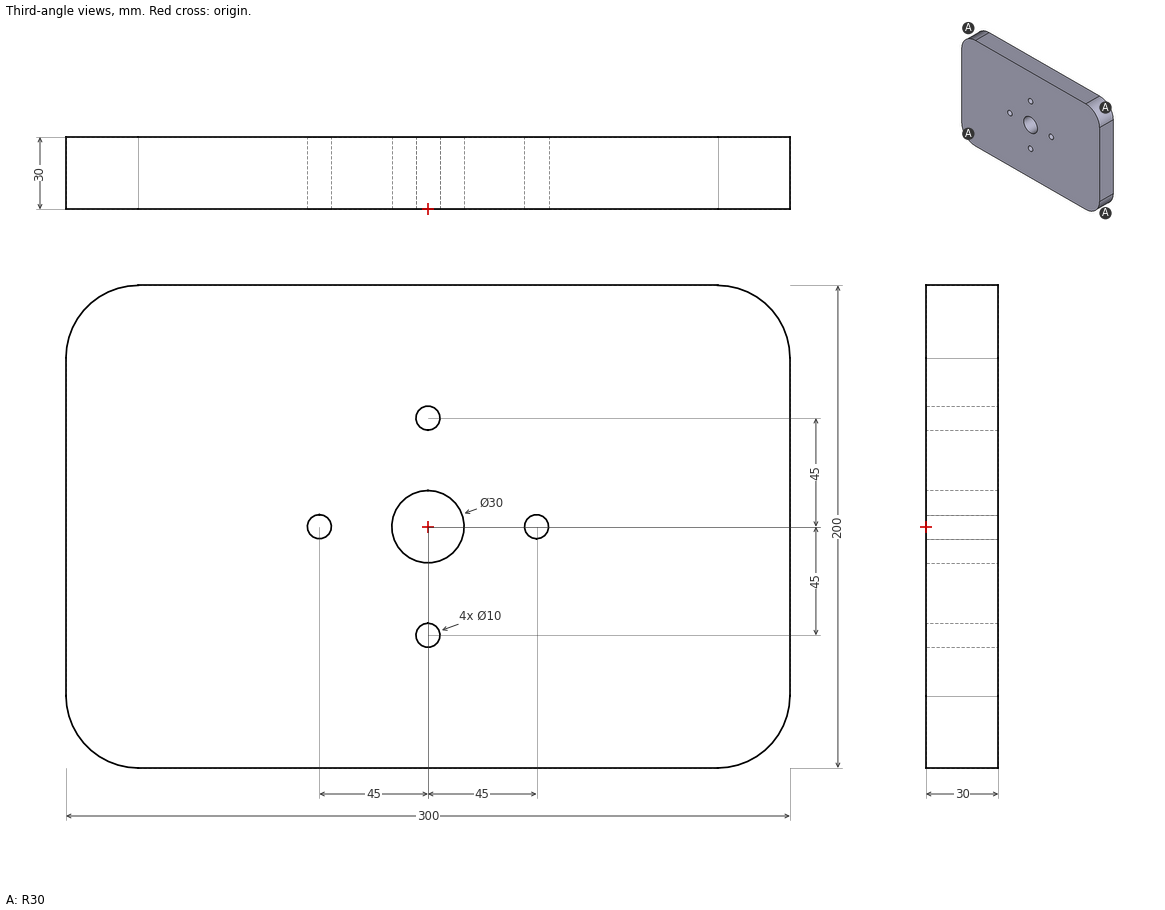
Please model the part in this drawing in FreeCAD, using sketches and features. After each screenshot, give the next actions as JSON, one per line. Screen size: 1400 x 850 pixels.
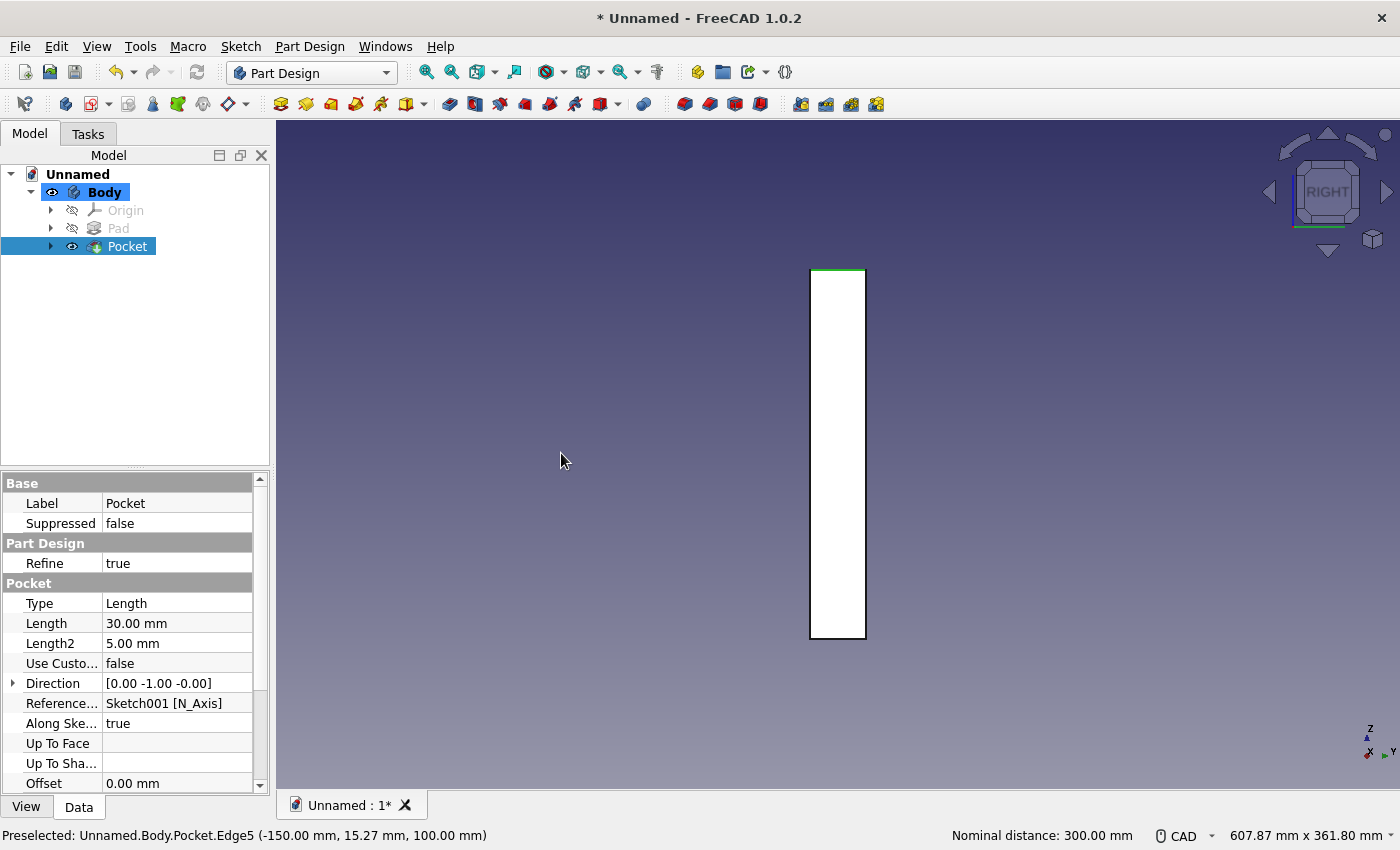
{"action": "left_click", "coordinate": [838, 638], "text": "ctrl"}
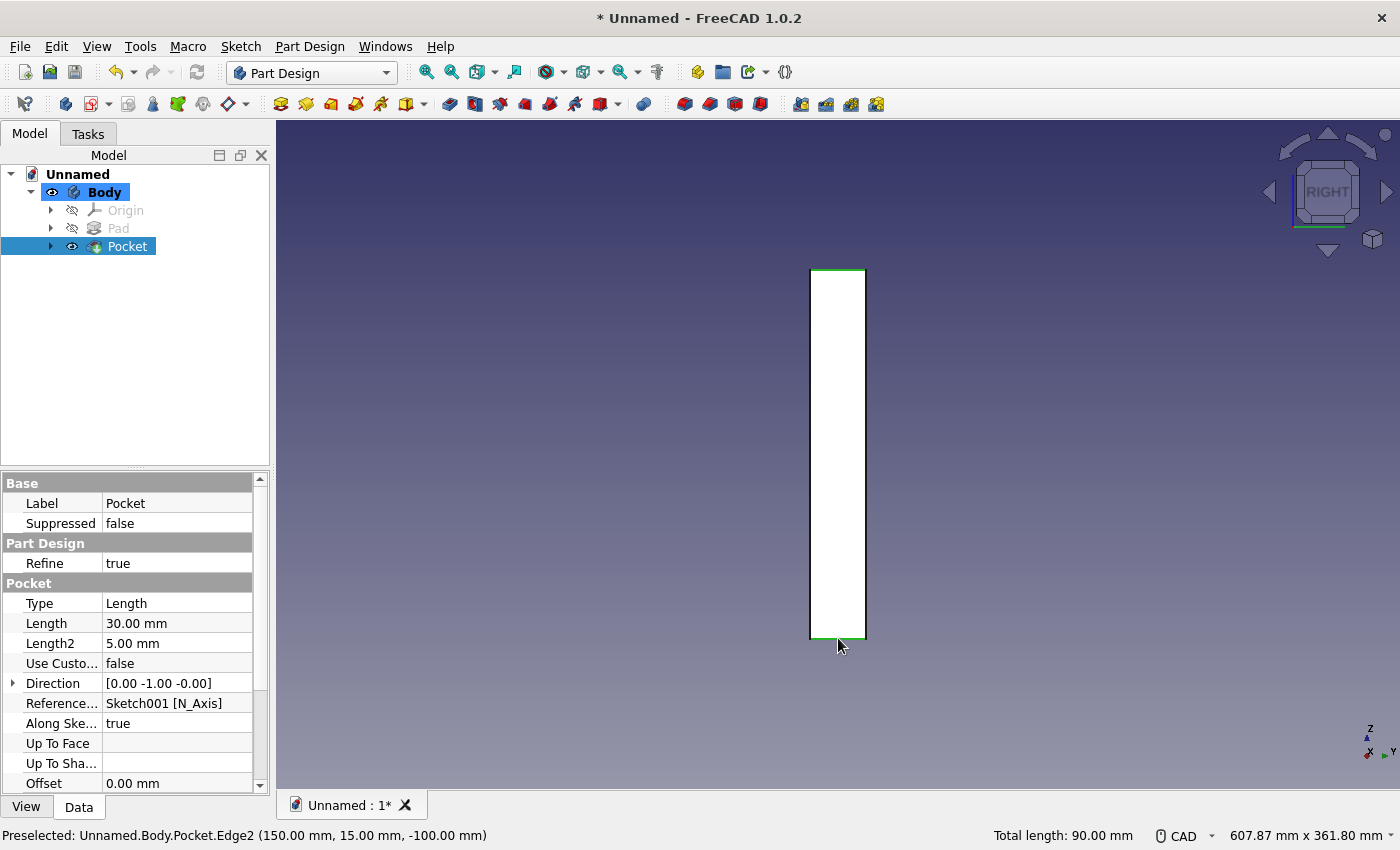
{"action": "key", "text": "5"}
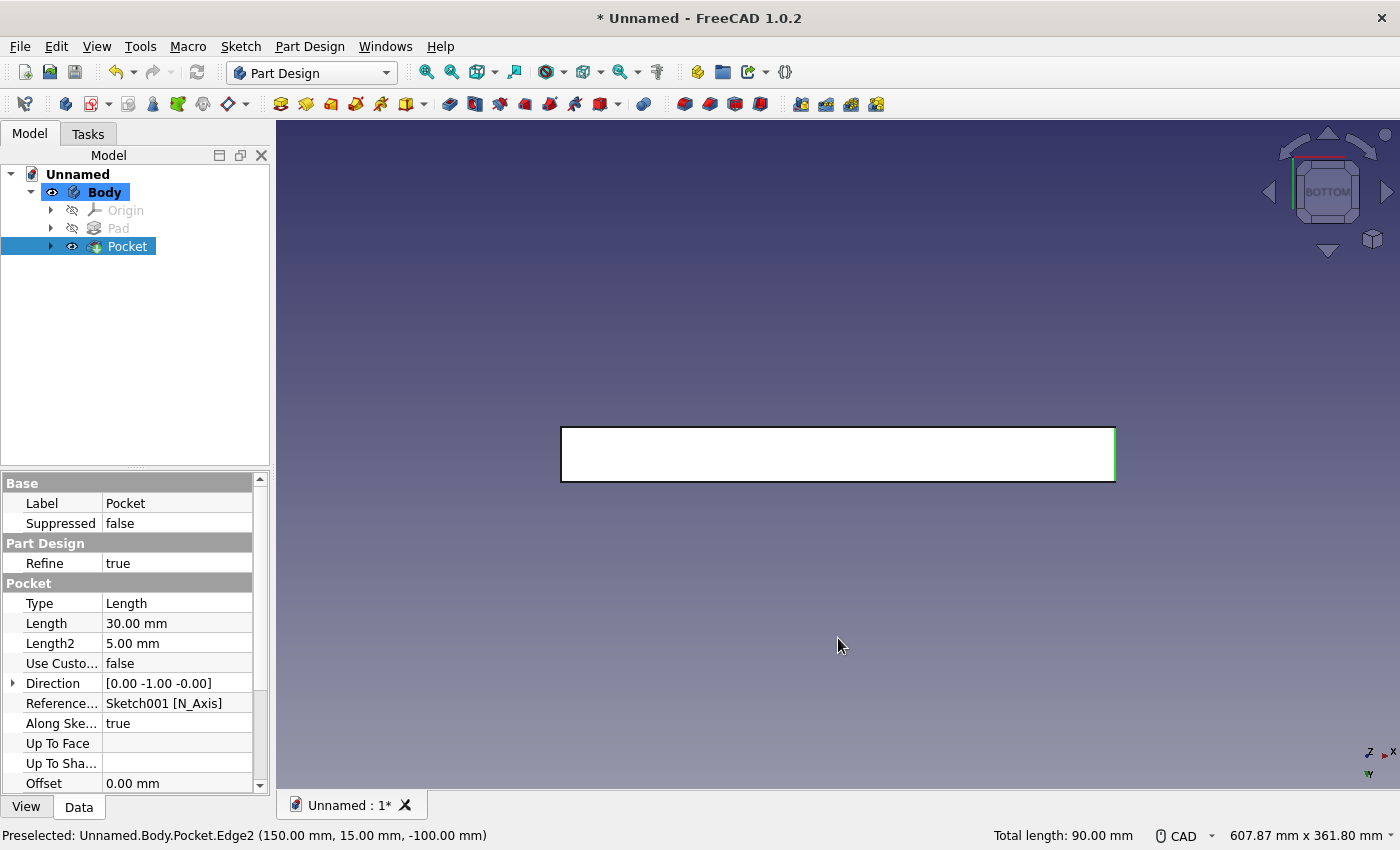
{"action": "left_click", "coordinate": [561, 454], "text": "ctrl"}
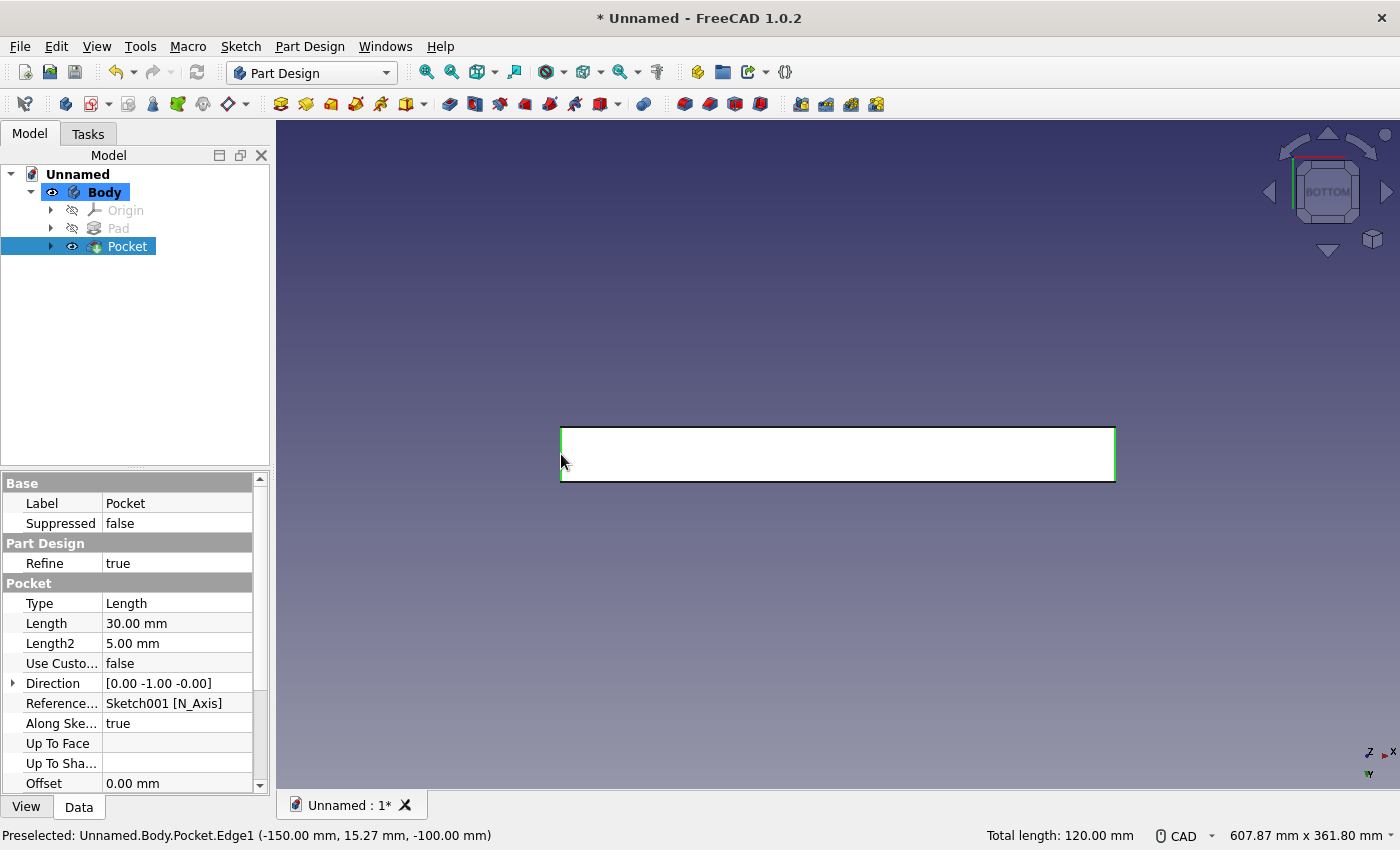
{"action": "left_click", "coordinate": [685, 104]}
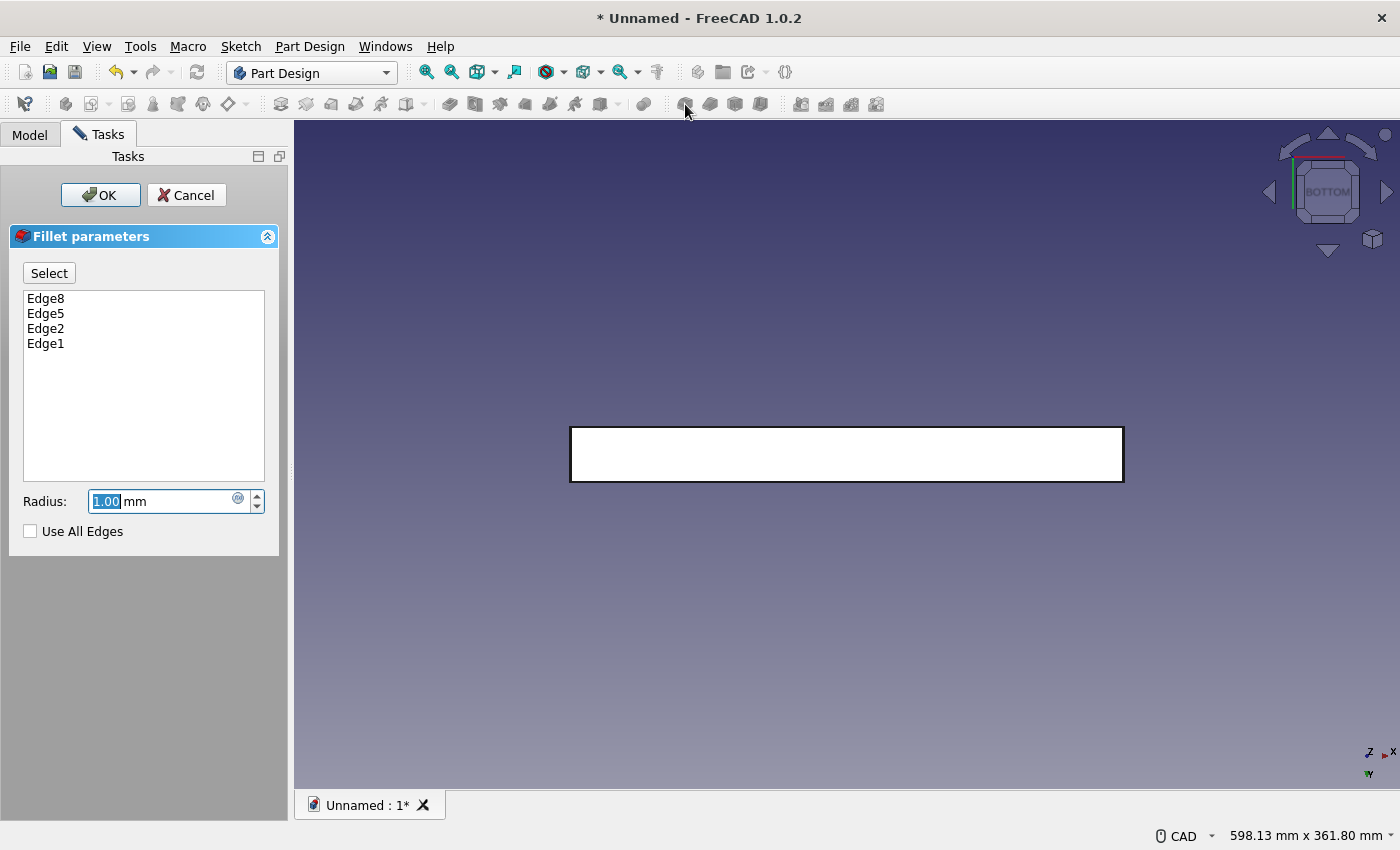
{"action": "type", "text": "30"}
{"action": "key", "text": "Tab"}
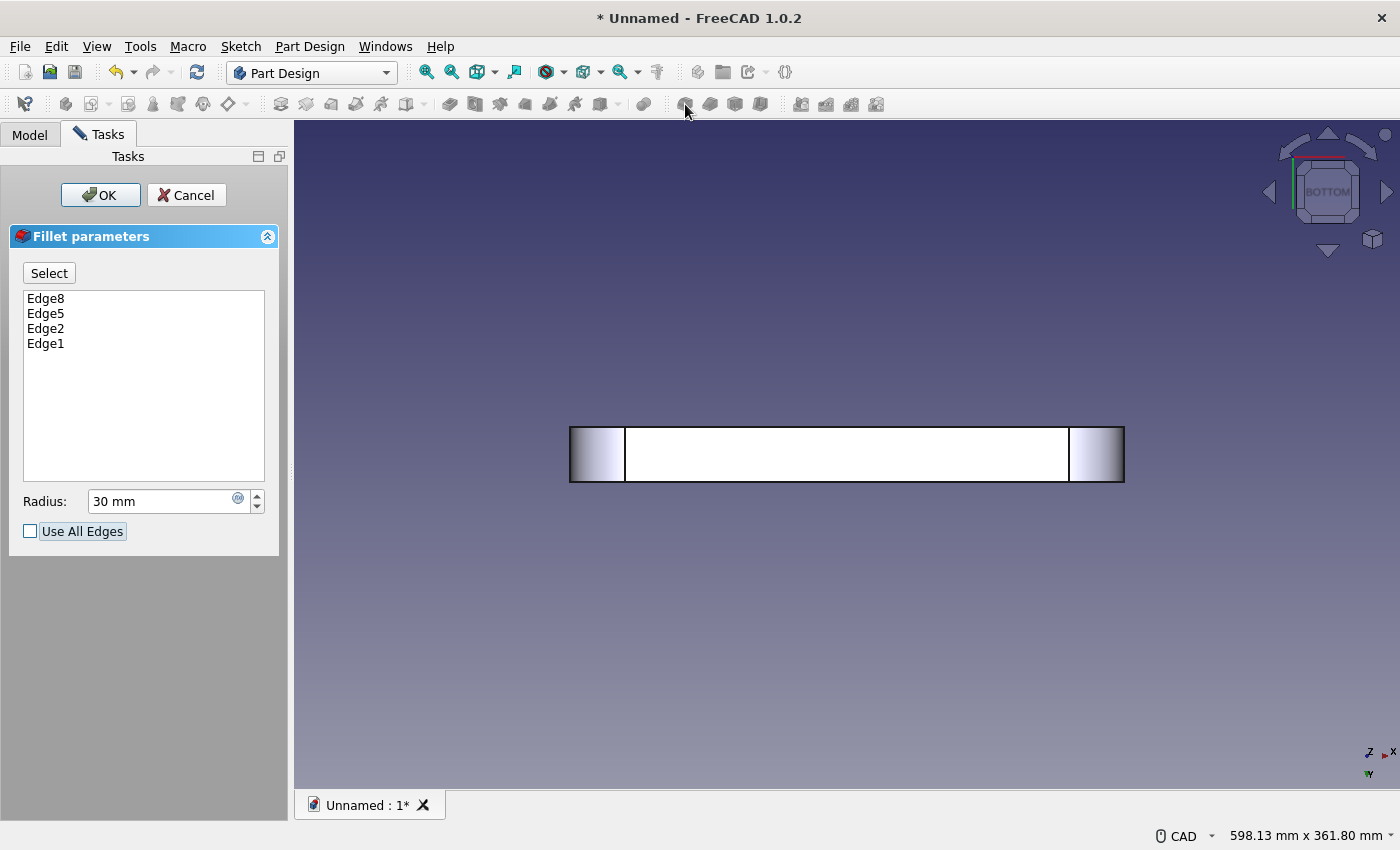
{"action": "left_click", "coordinate": [101, 195]}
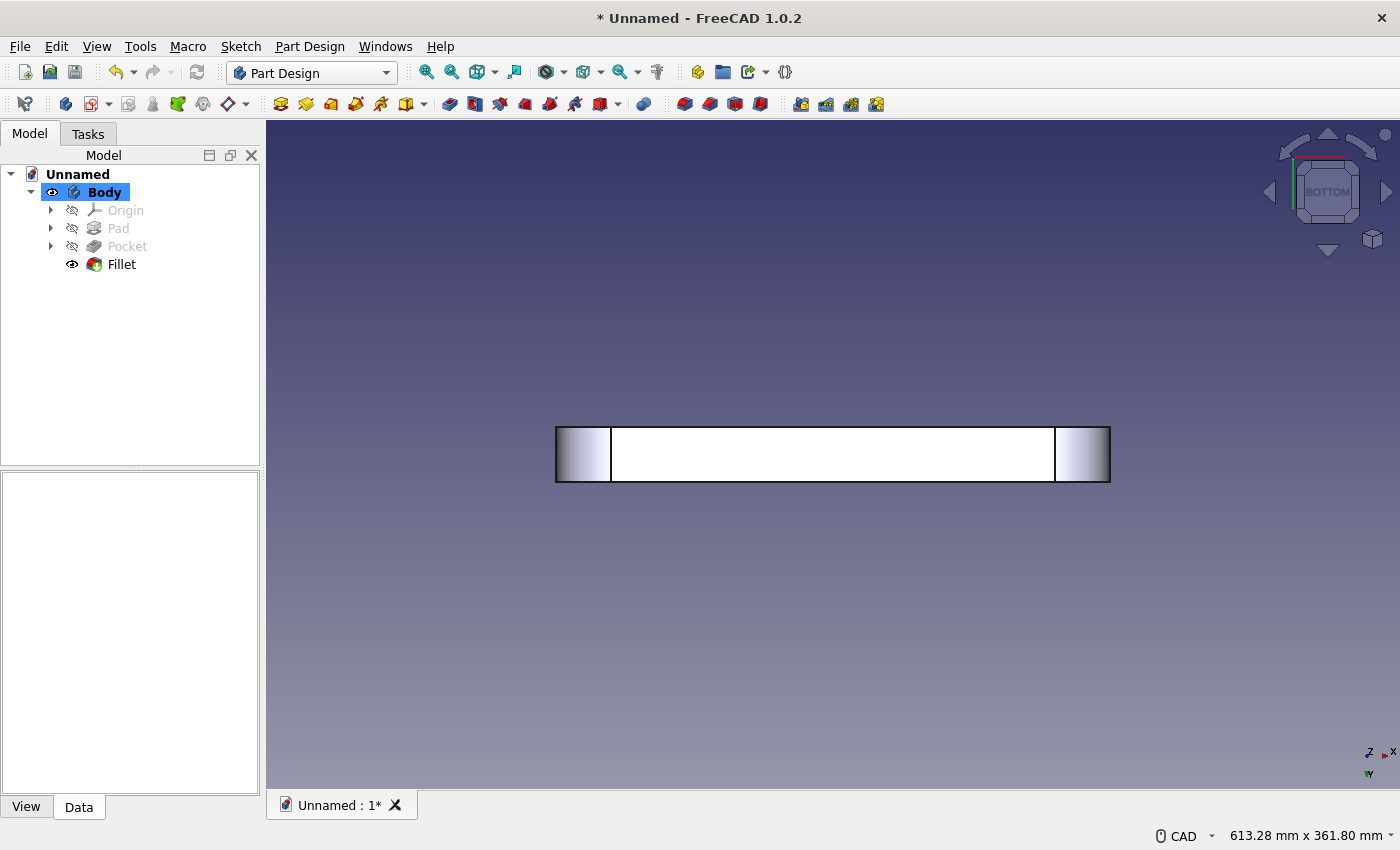
{"action": "key", "text": "0"}